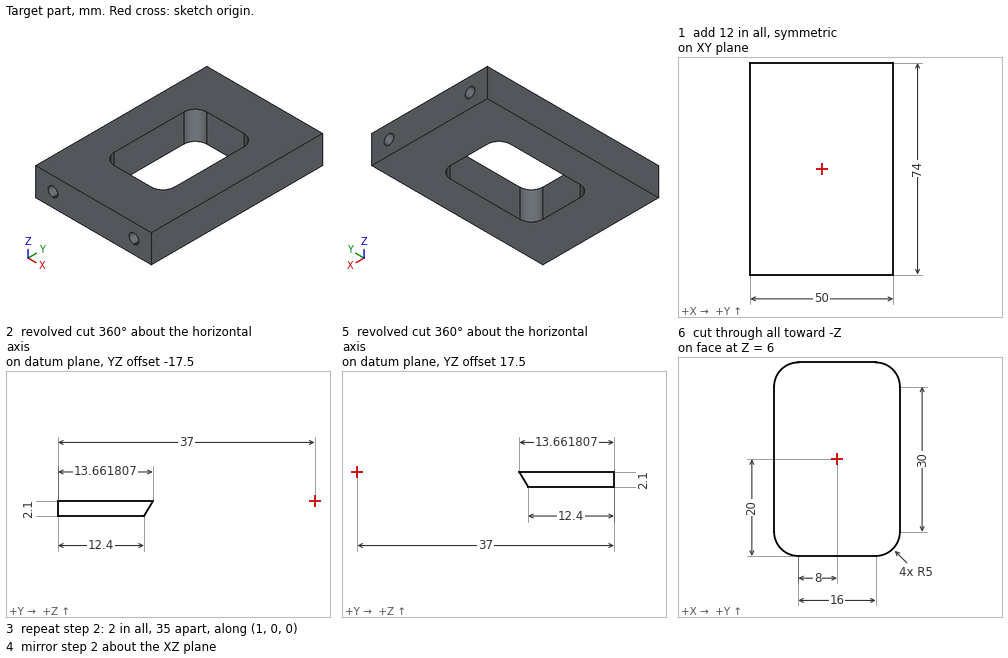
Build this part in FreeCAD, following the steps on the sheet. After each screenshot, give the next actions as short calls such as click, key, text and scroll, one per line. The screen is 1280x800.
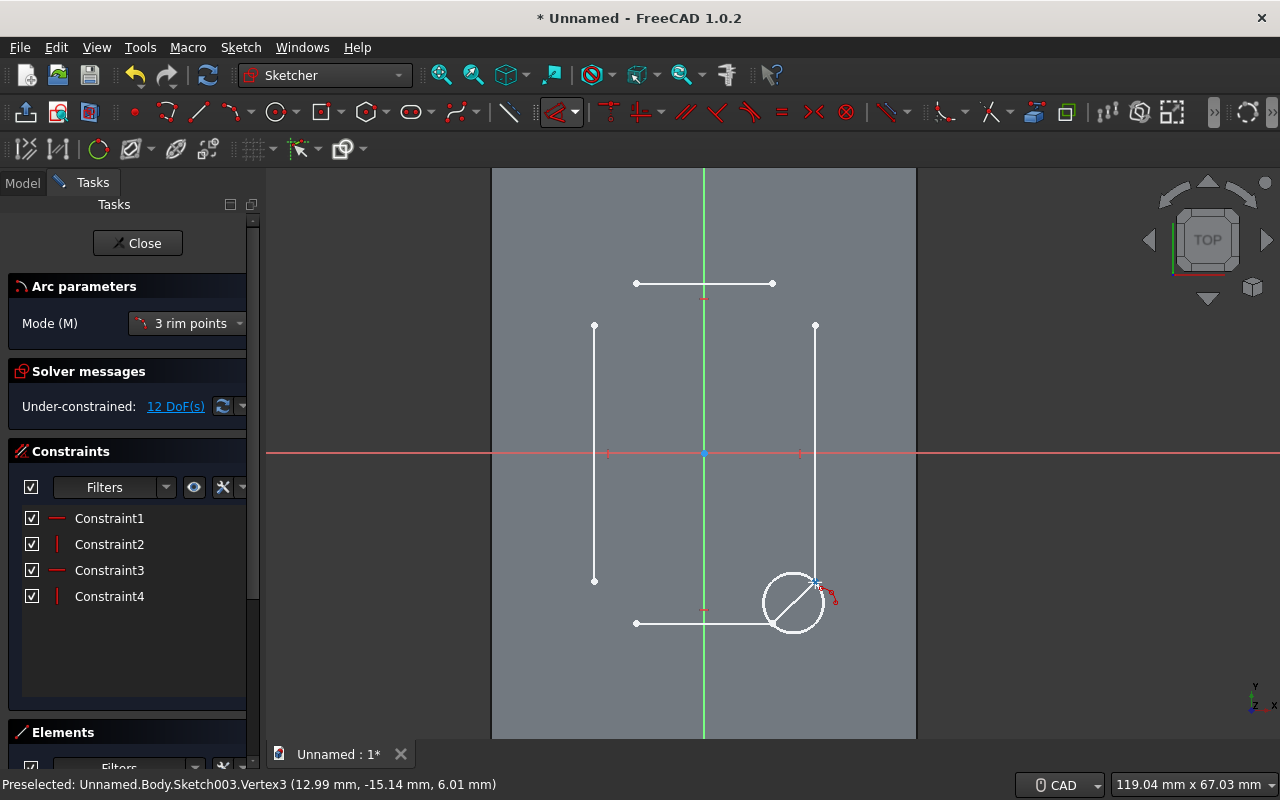
scroll(803, 611, up, 2)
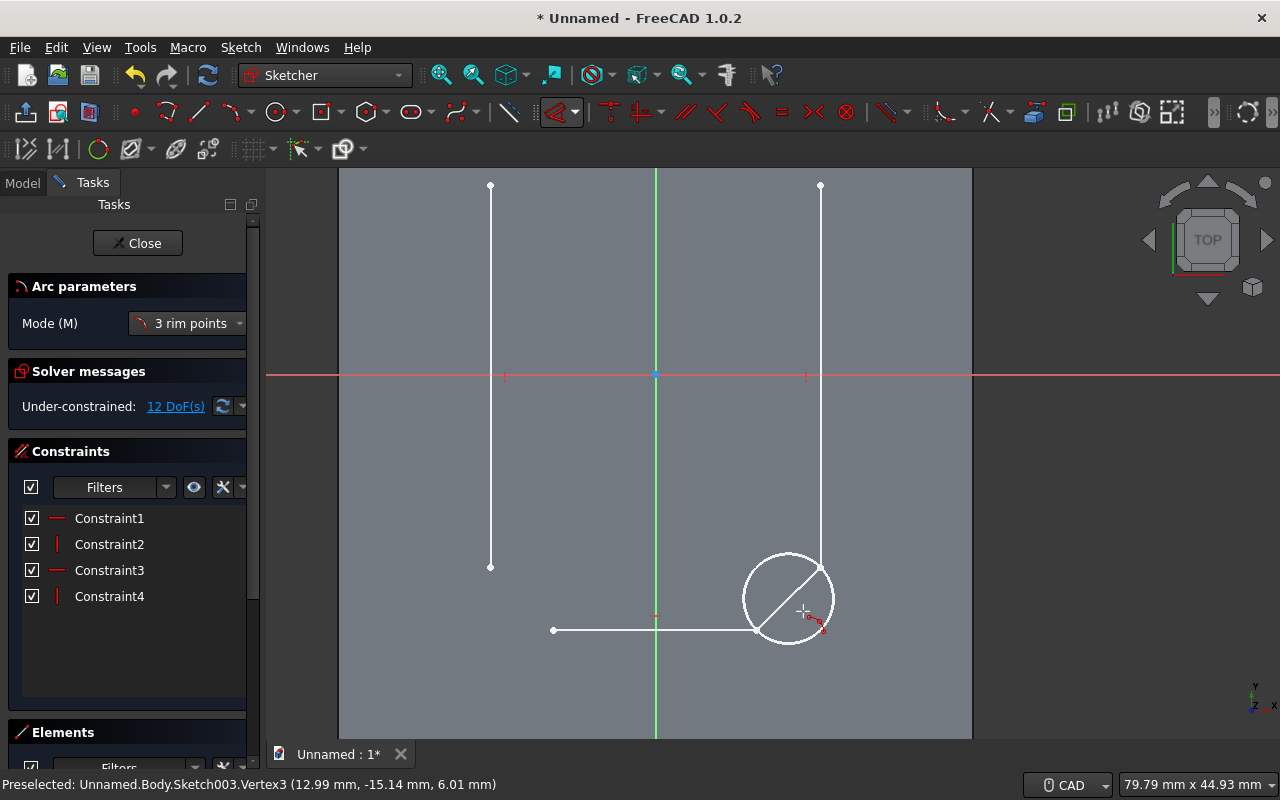
click(802, 610)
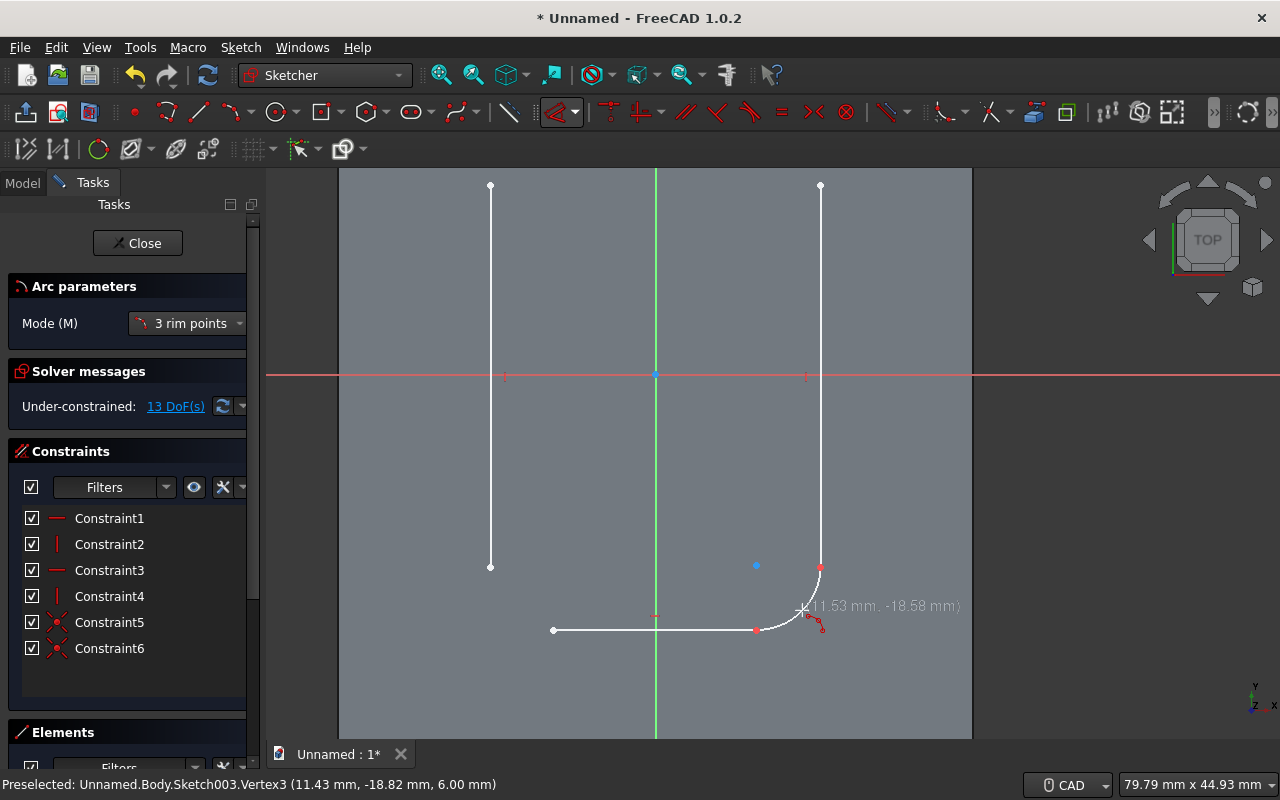
scroll(804, 613, down, 2)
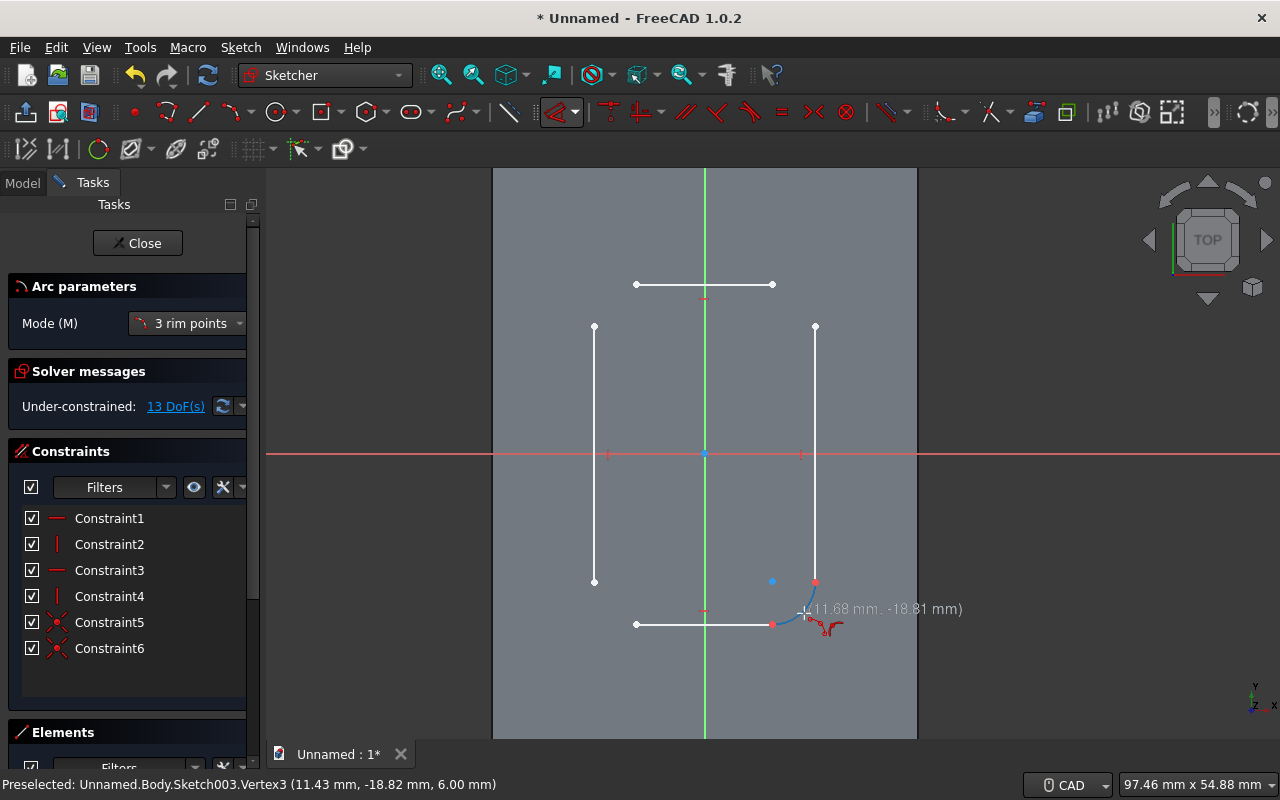
click(815, 327)
click(772, 285)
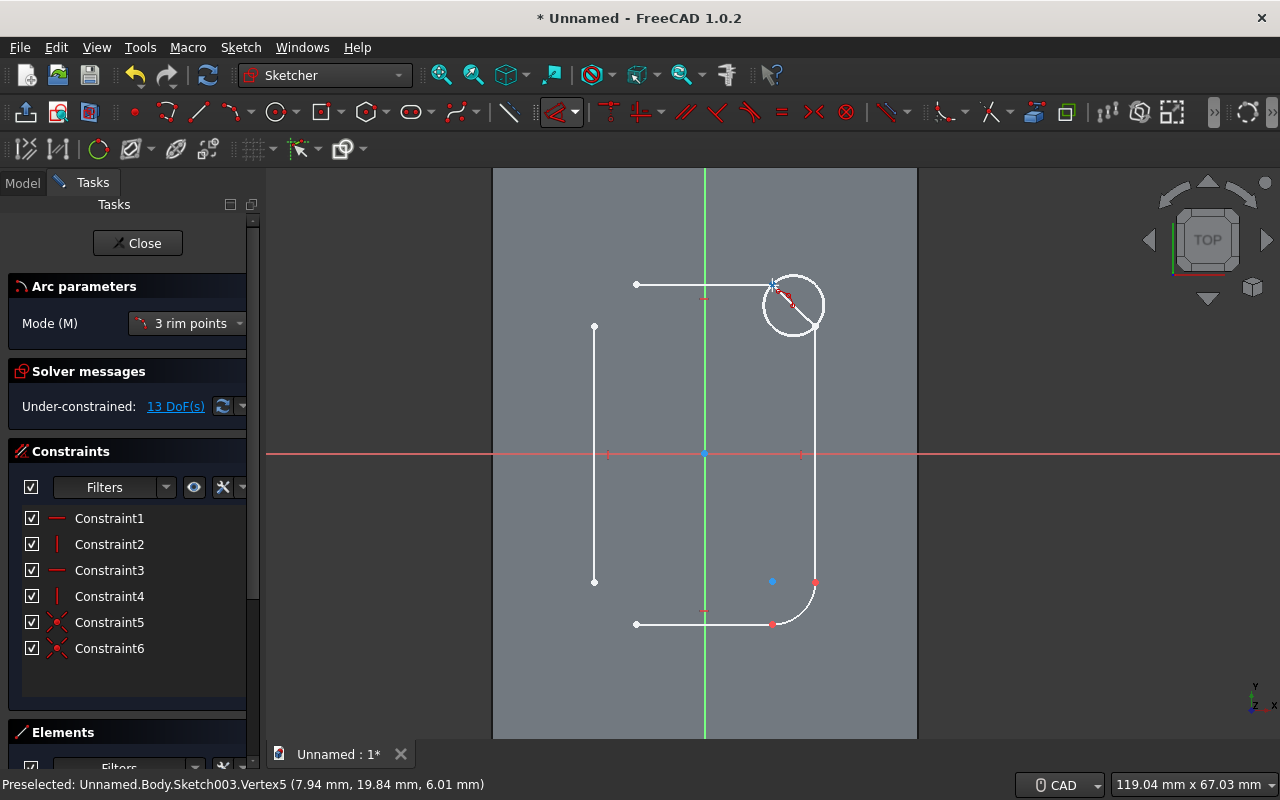
scroll(803, 296, up, 2)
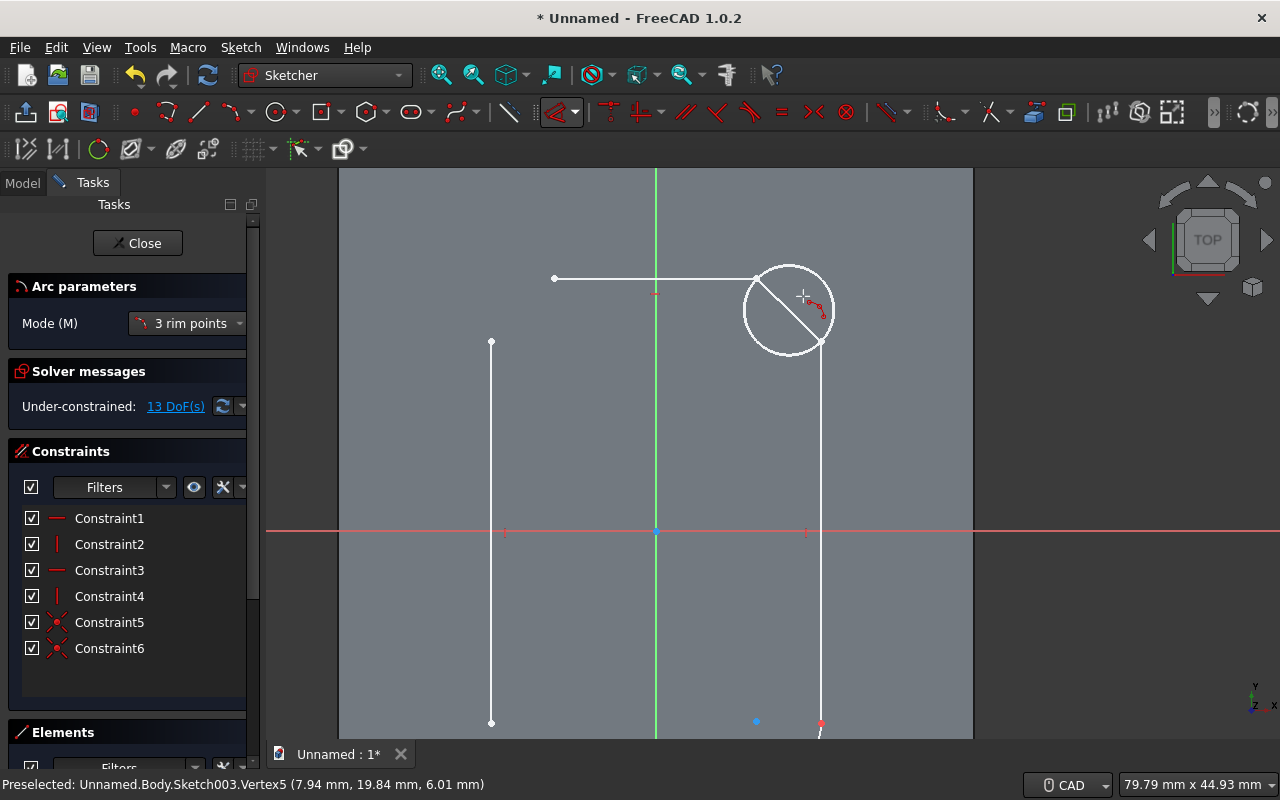
click(803, 296)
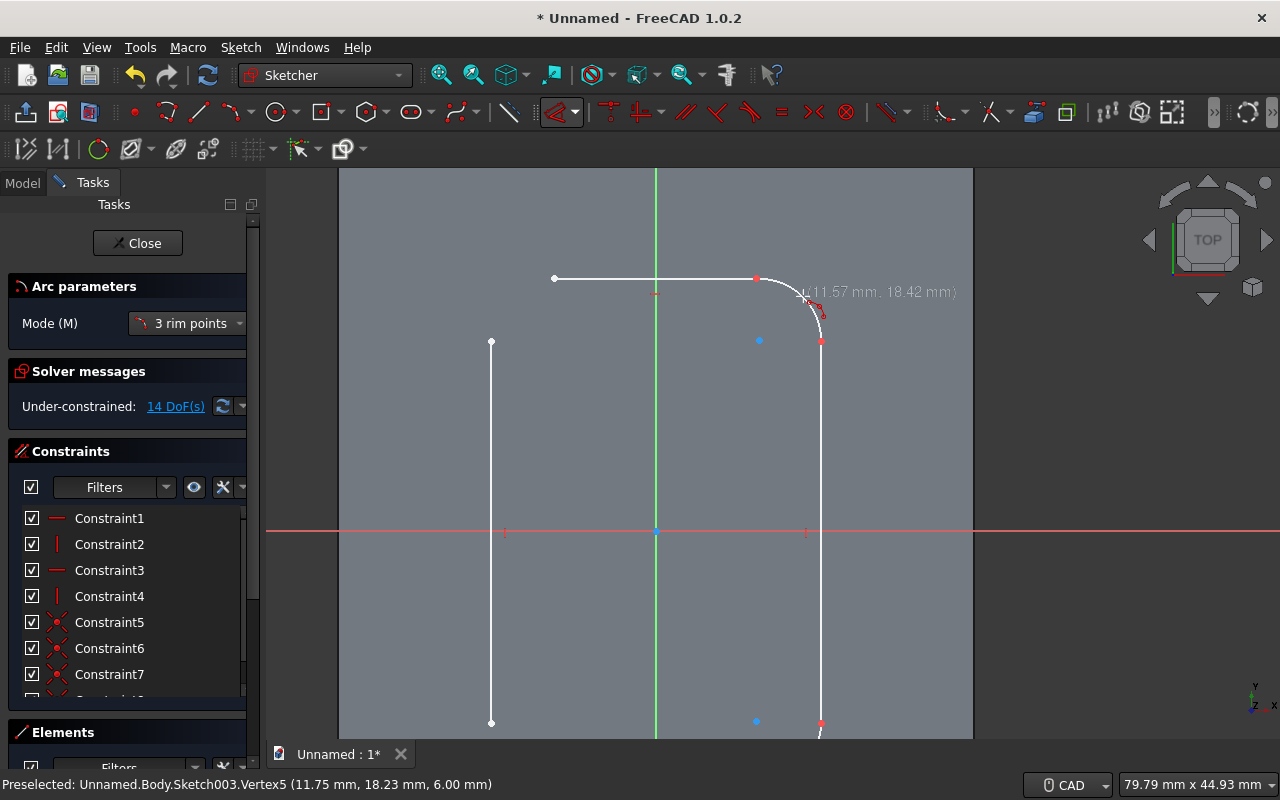
click(554, 279)
click(491, 342)
click(509, 296)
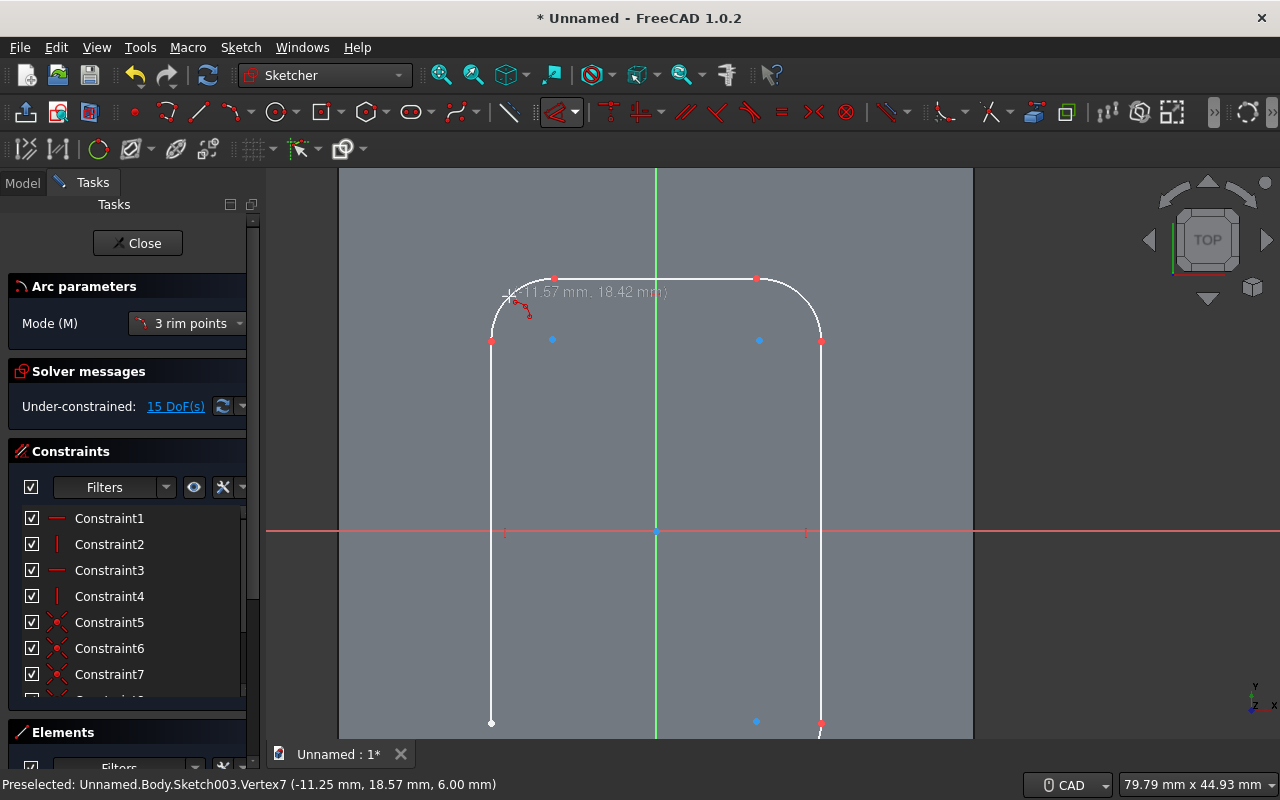
scroll(803, 296, down, 2)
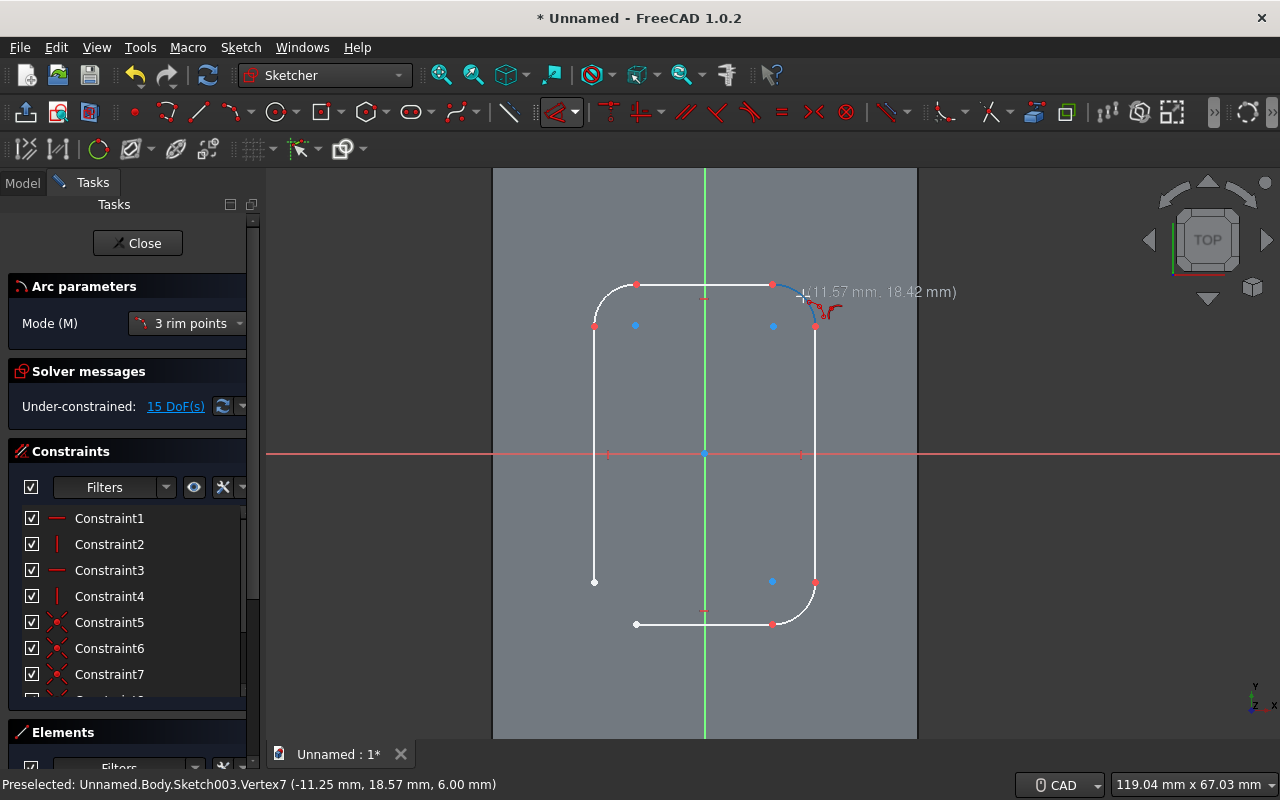
click(594, 583)
click(636, 625)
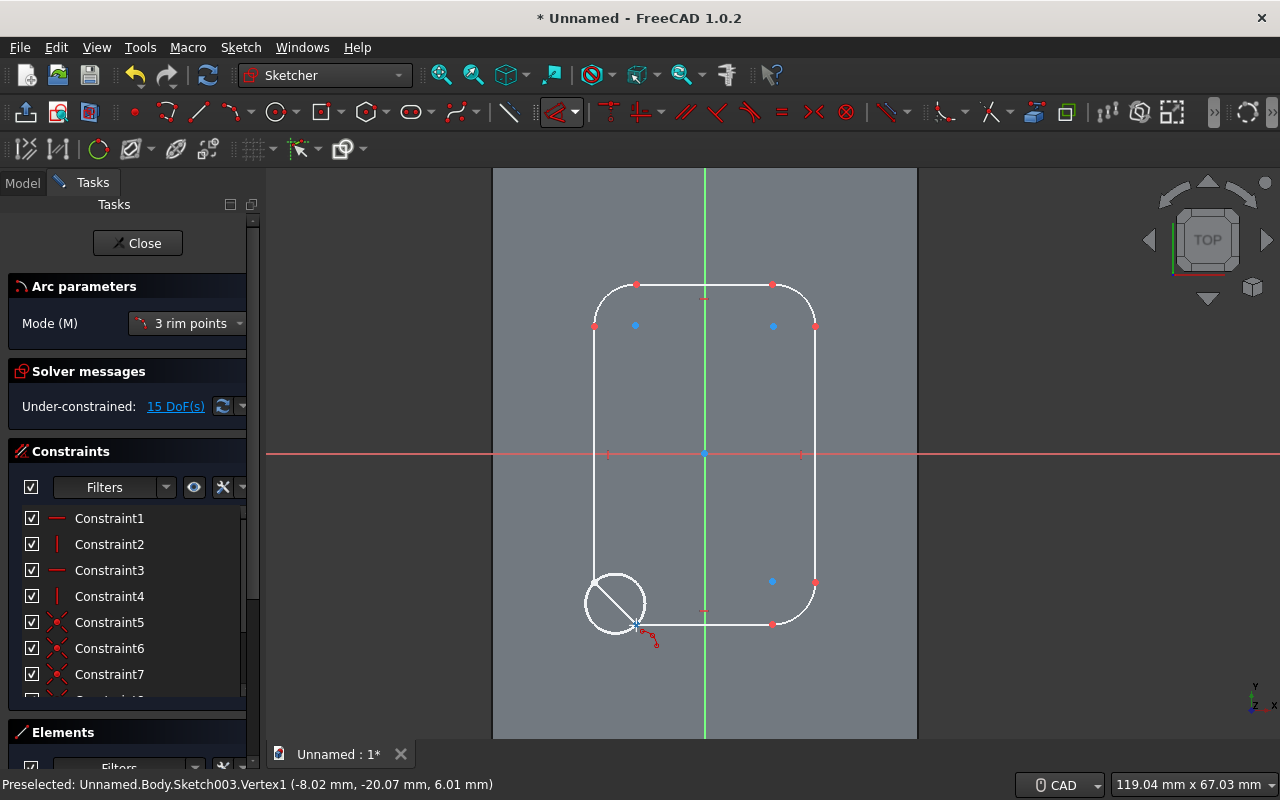
scroll(606, 612, up, 2)